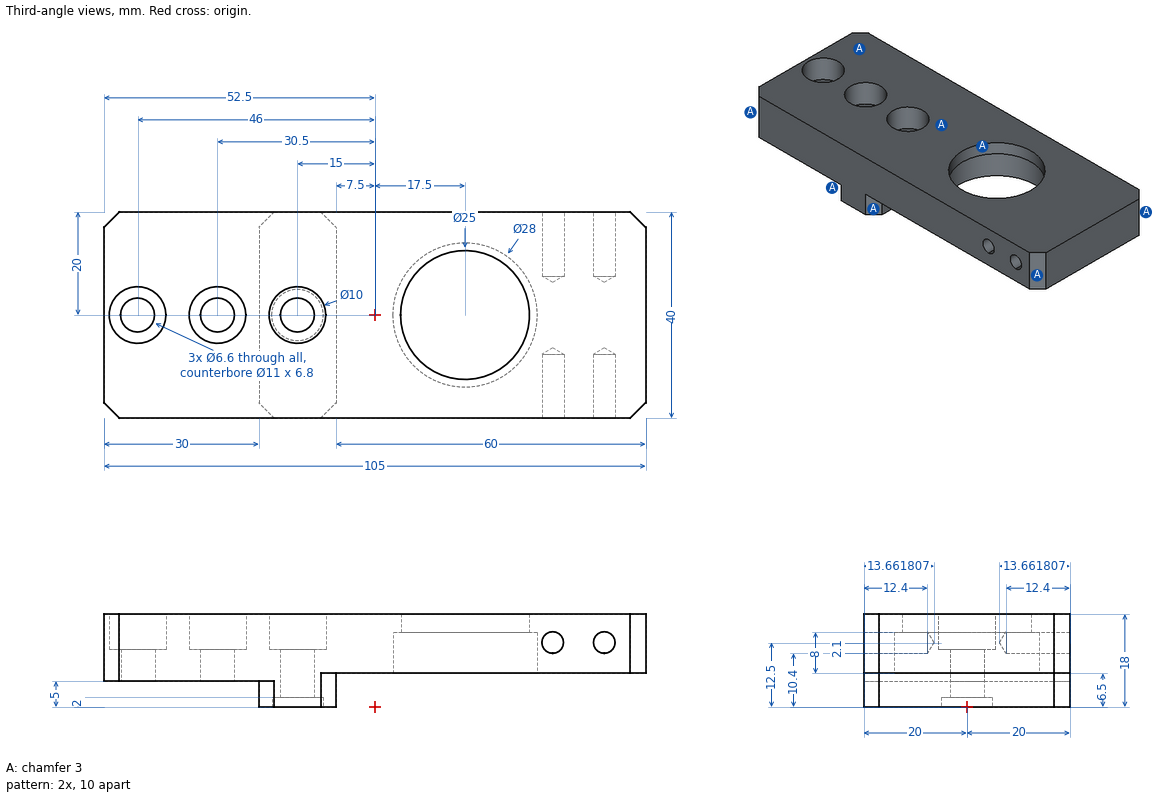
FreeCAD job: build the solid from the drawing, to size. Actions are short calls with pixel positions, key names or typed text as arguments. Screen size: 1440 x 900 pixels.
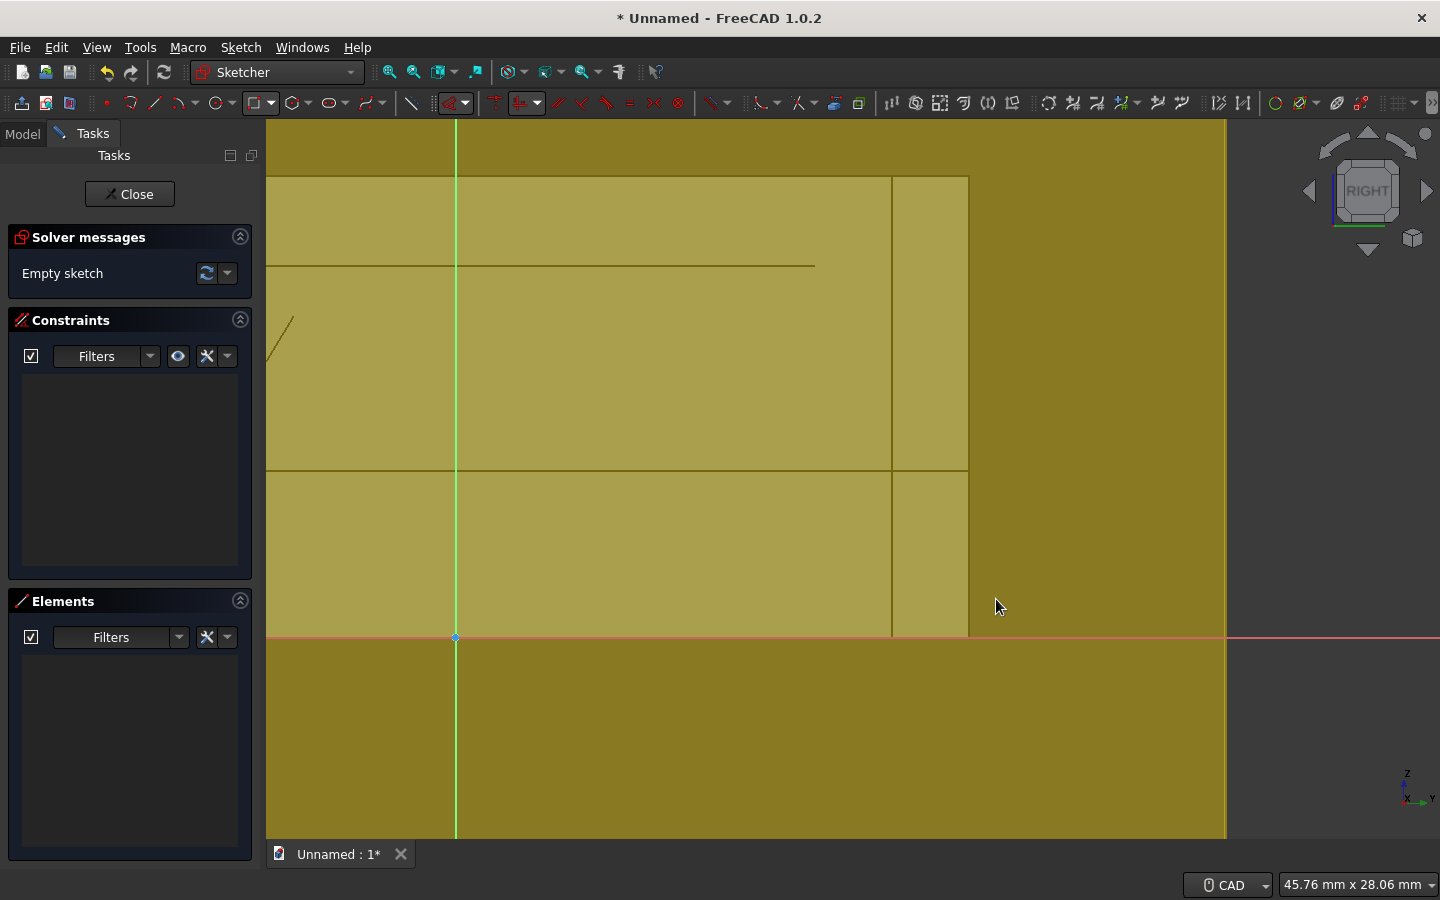
click(132, 104)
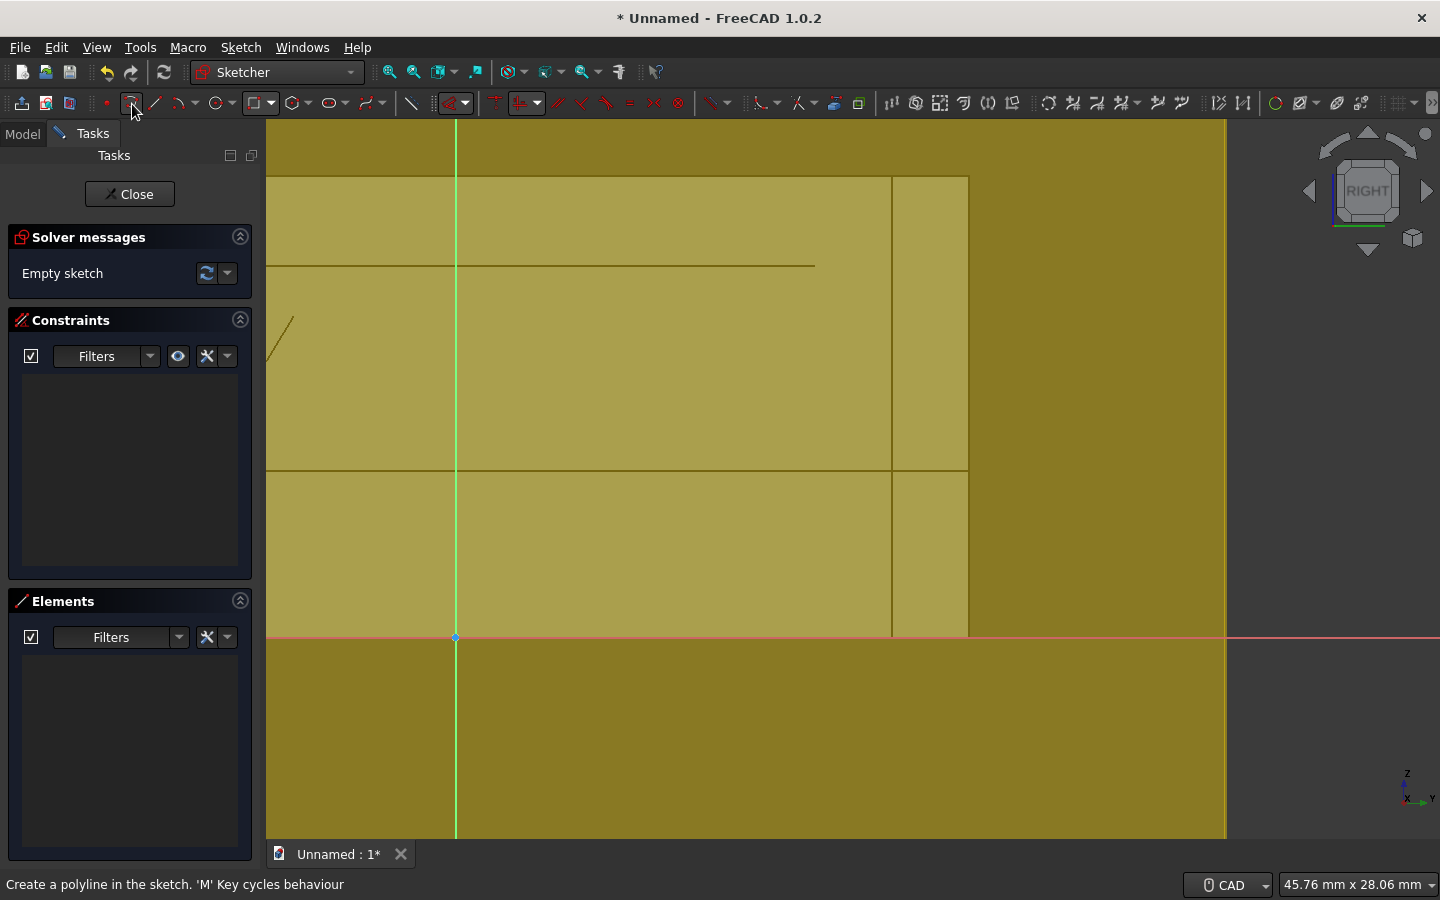
click(651, 371)
click(969, 371)
click(969, 317)
click(618, 317)
click(651, 372)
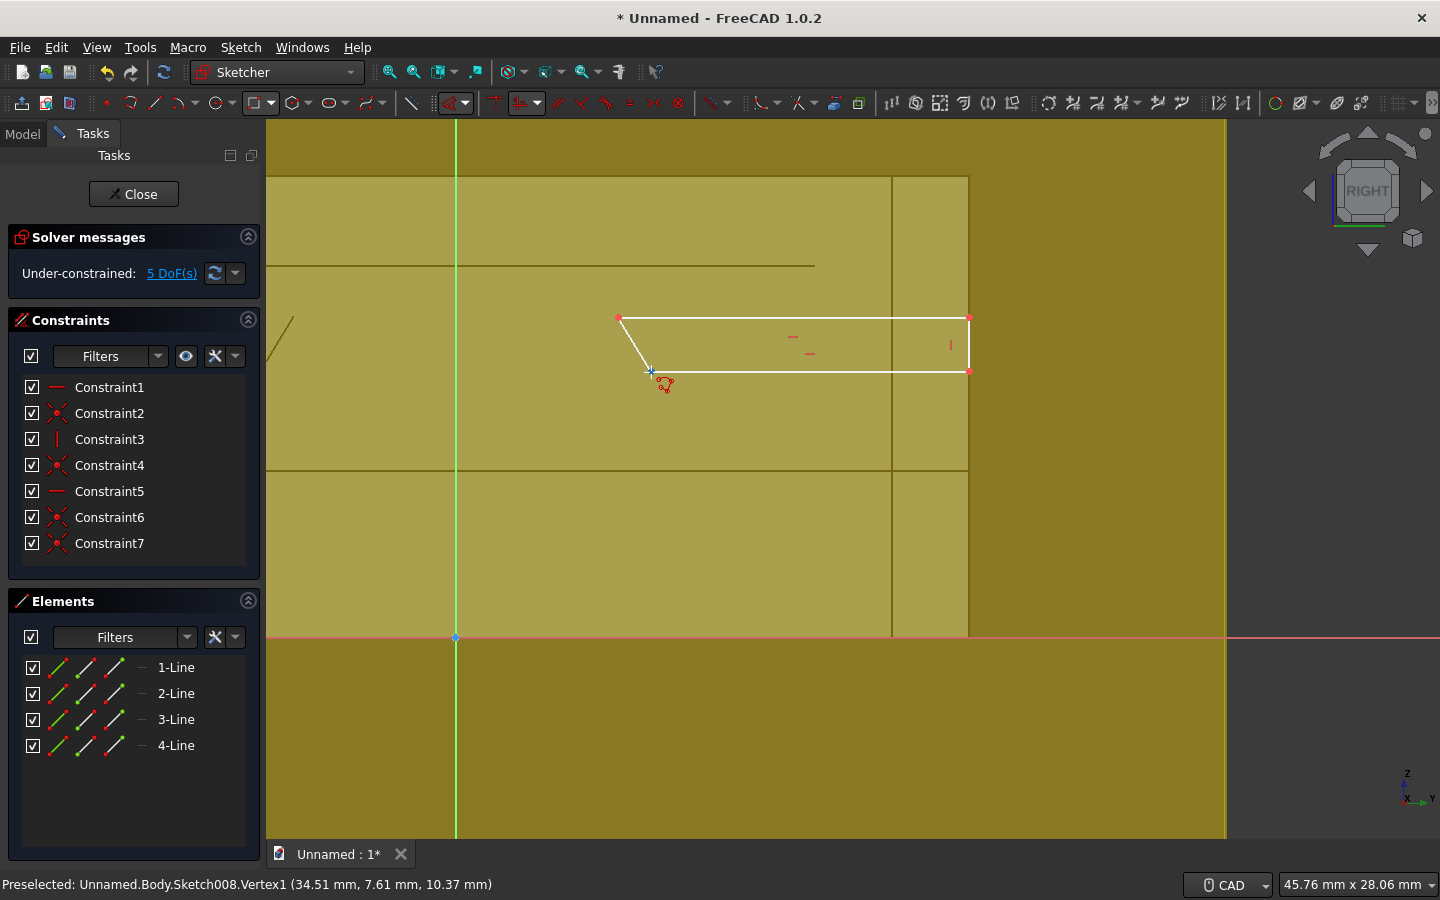
click(156, 104)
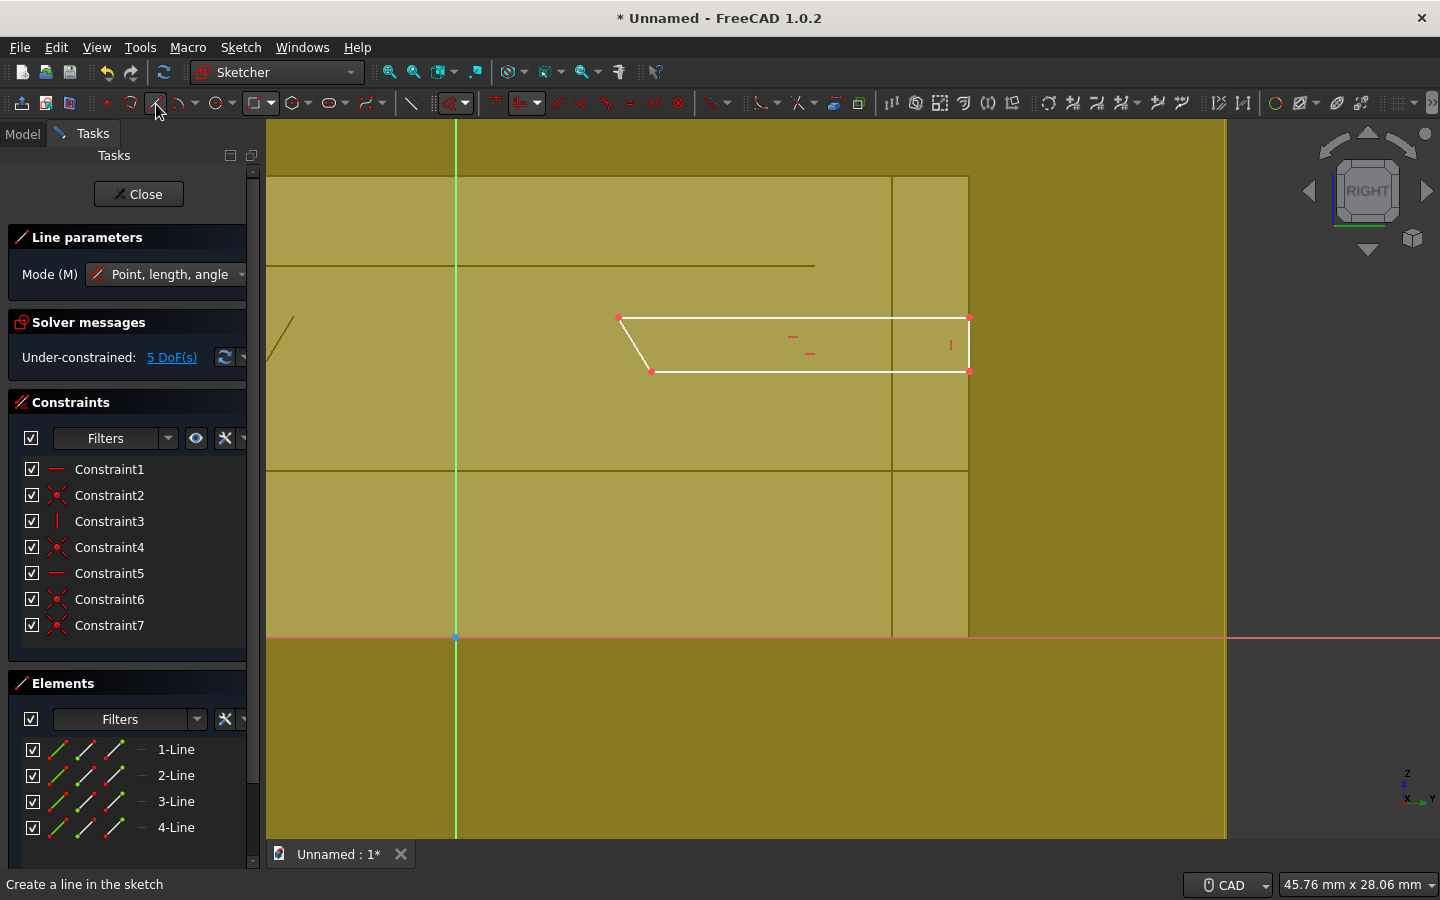
click(1004, 317)
click(1109, 317)
key(Escape)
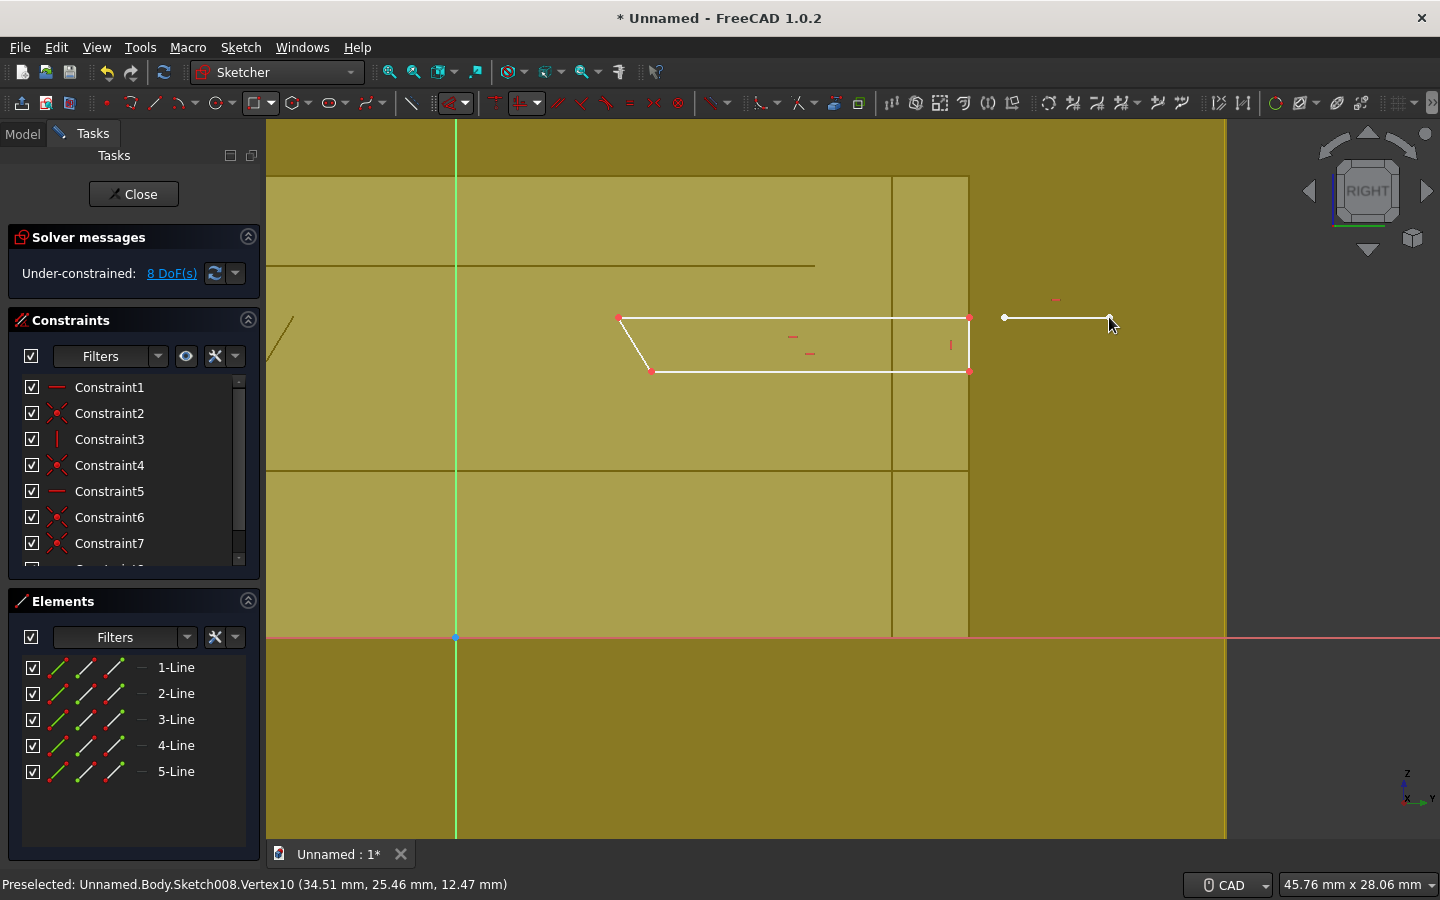
click(1035, 318)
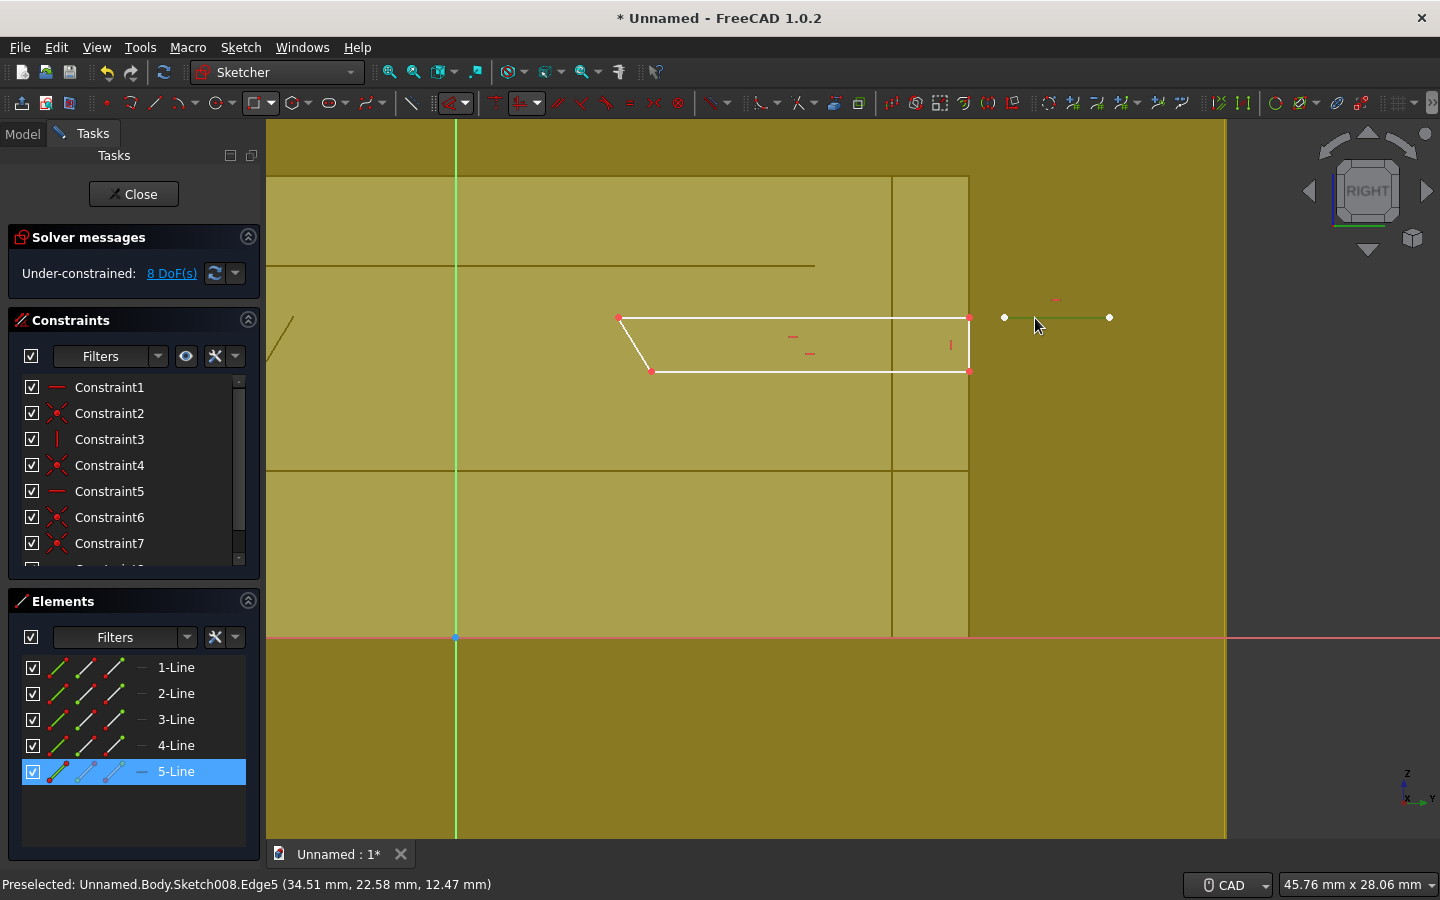
click(412, 104)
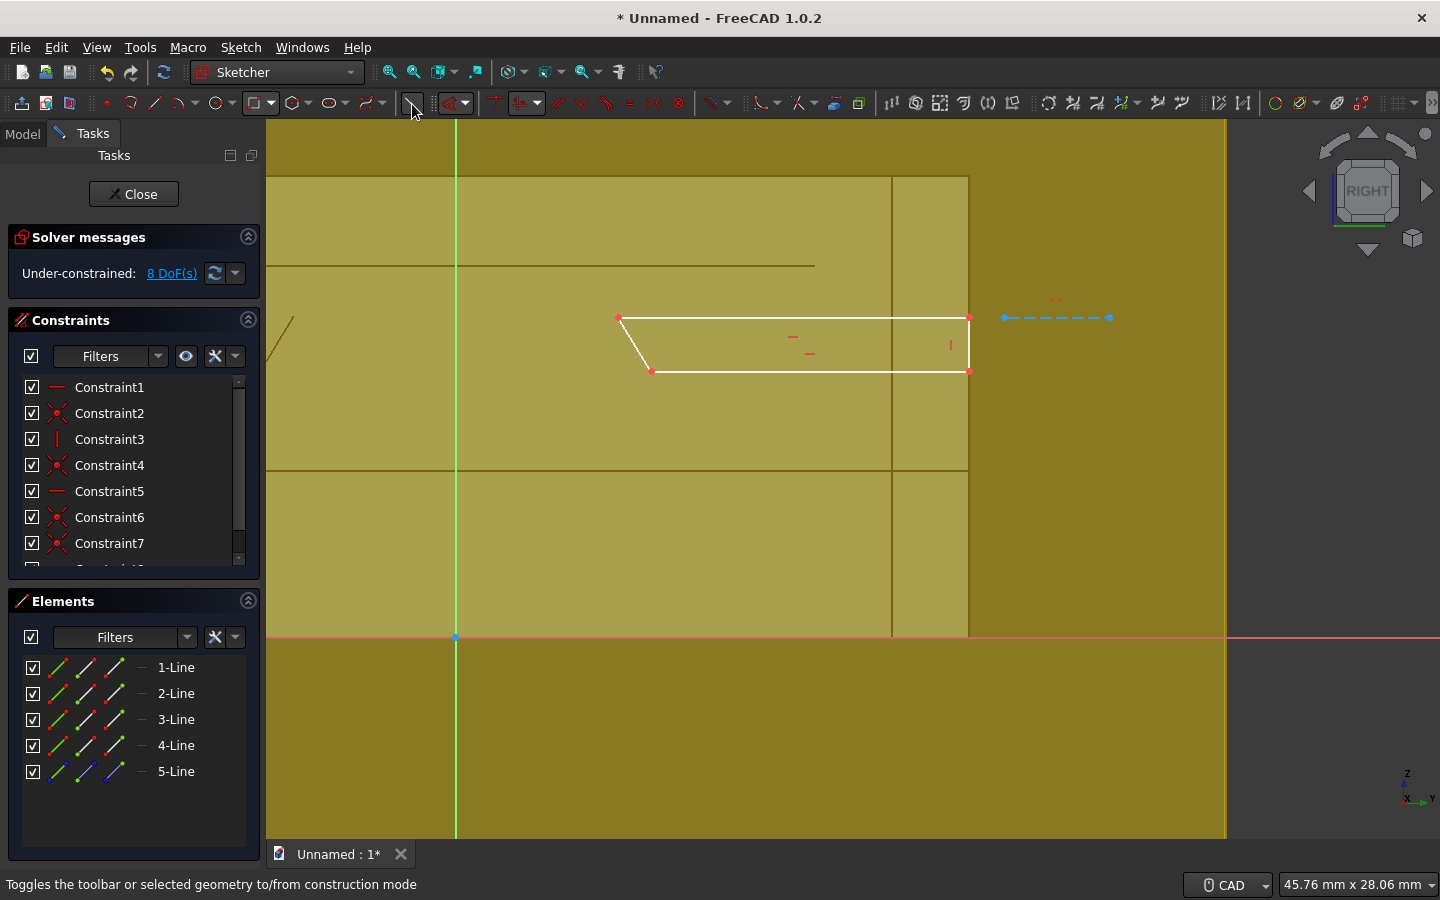
click(969, 356)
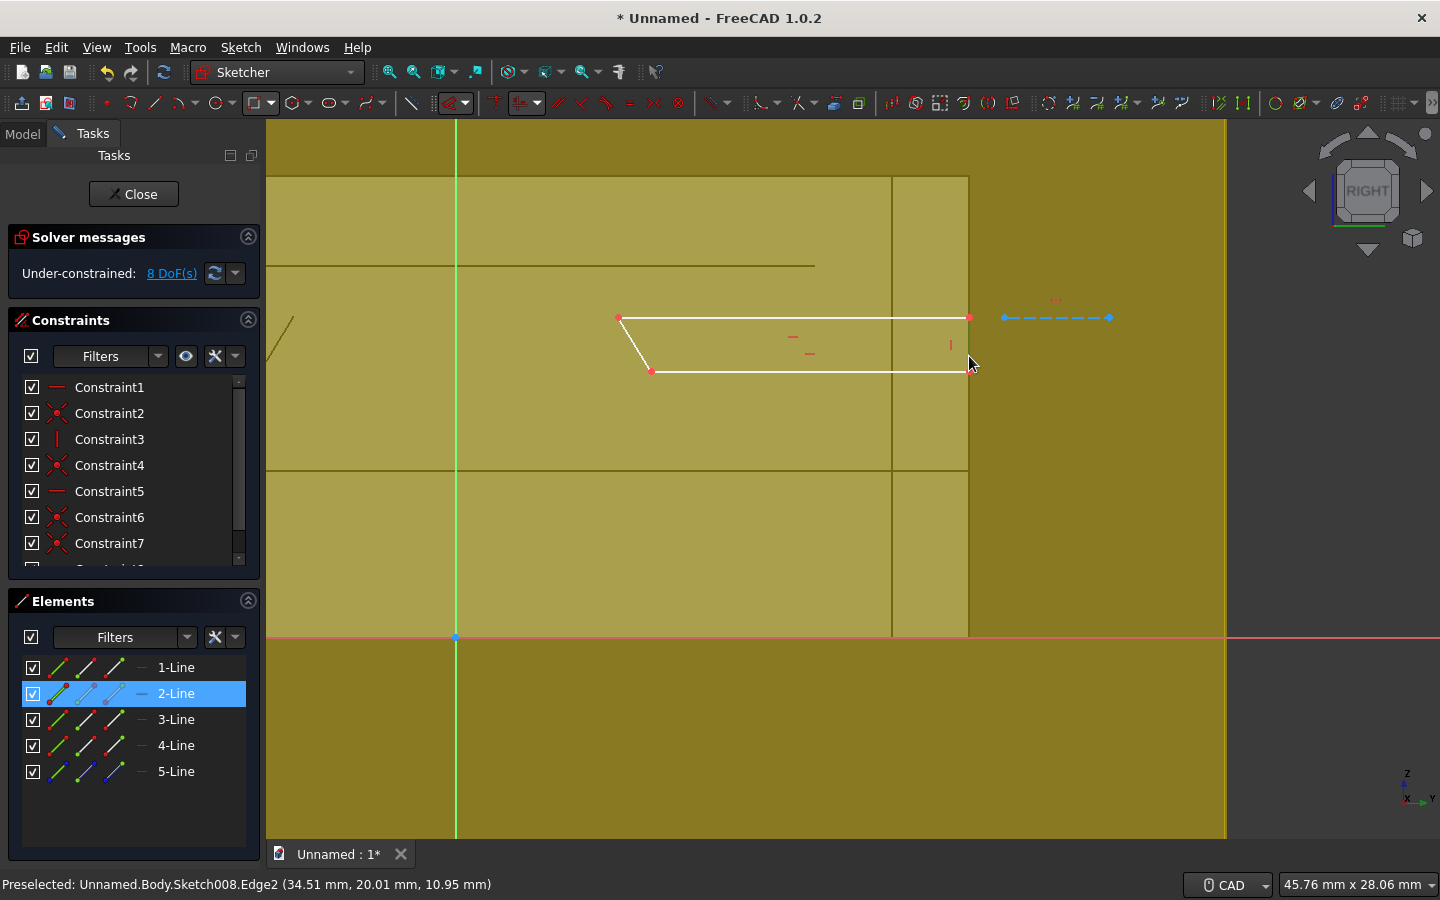
click(468, 104)